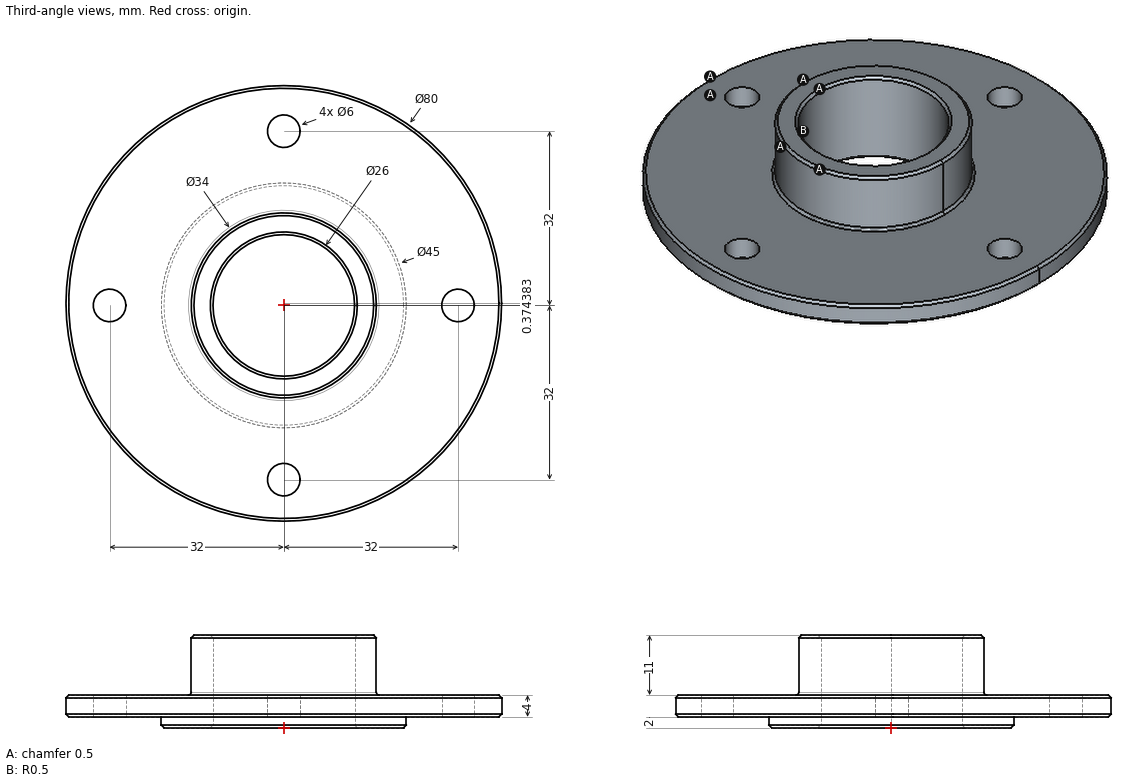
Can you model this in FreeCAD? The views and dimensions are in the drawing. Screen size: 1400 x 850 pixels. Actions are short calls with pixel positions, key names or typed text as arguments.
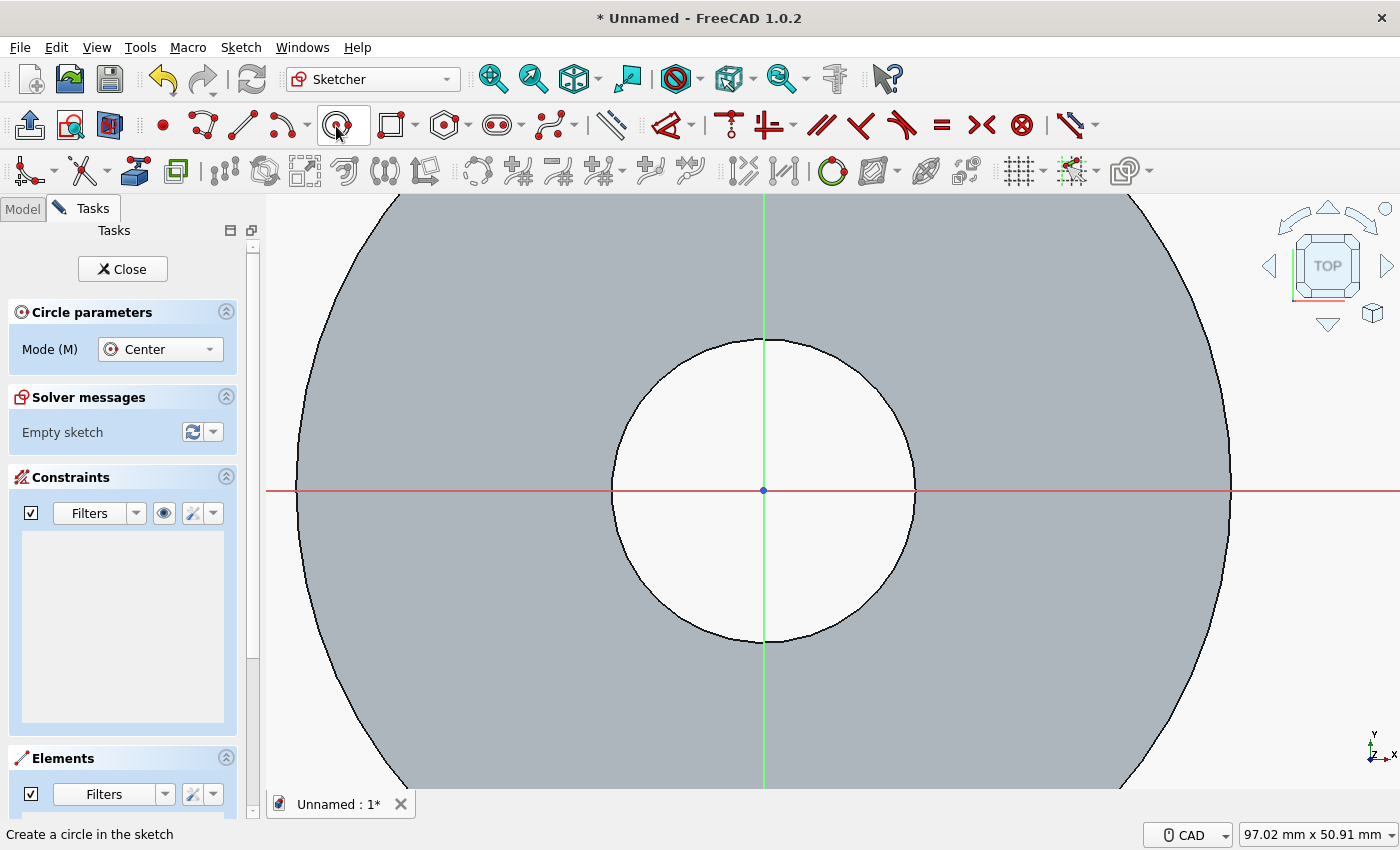
click(764, 491)
move(904, 350)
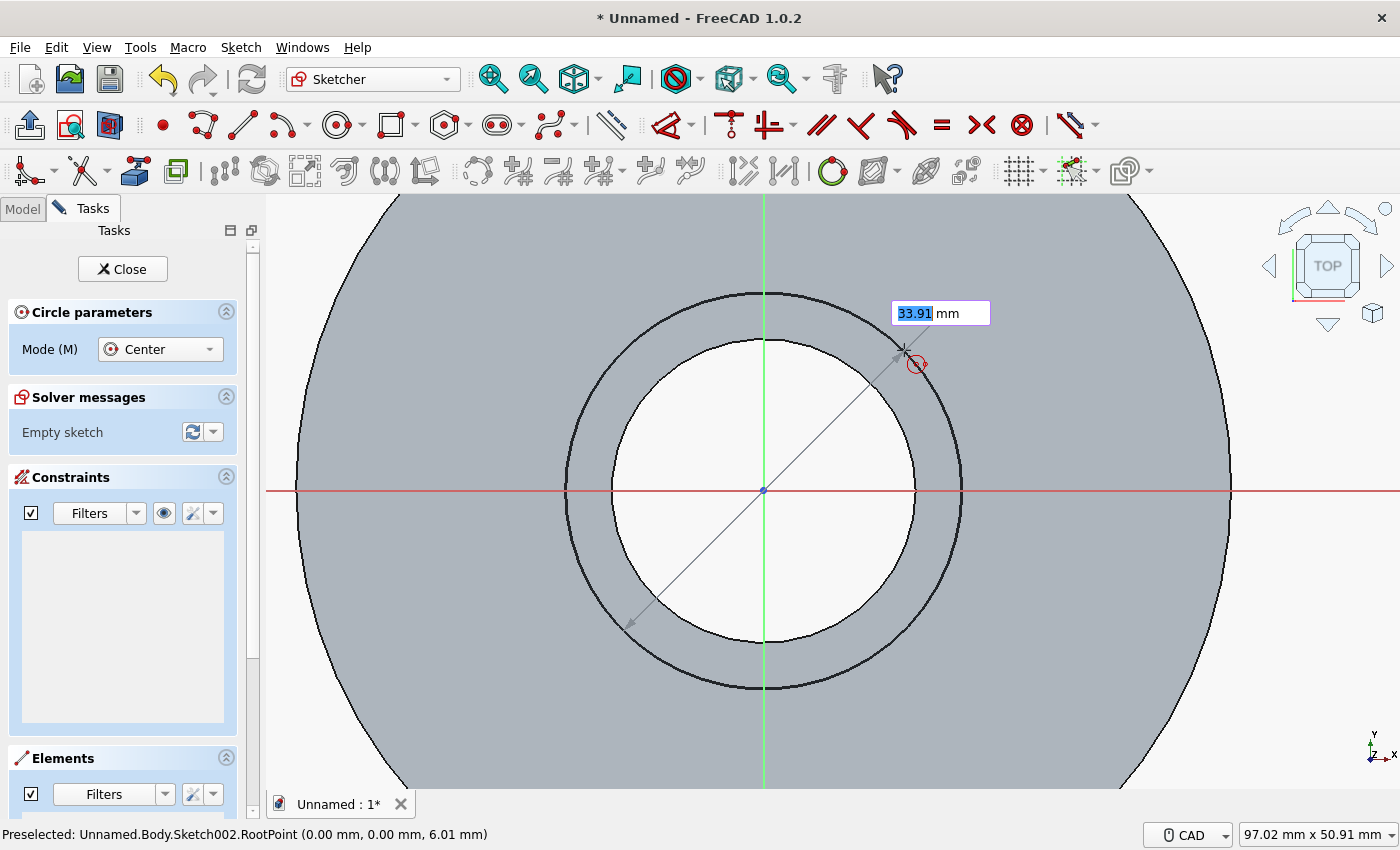
text(34)
key(Return)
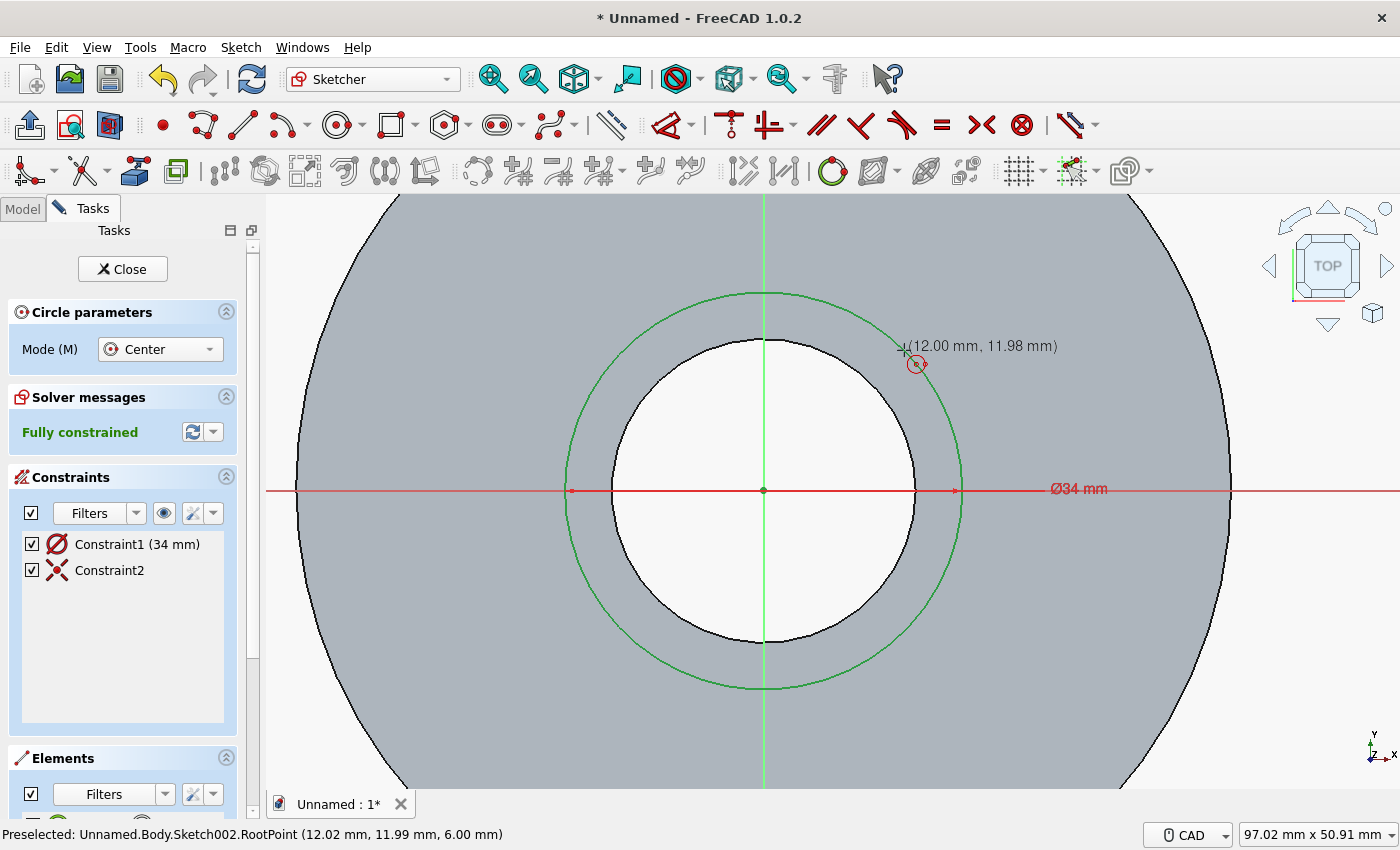
click(764, 491)
move(871, 384)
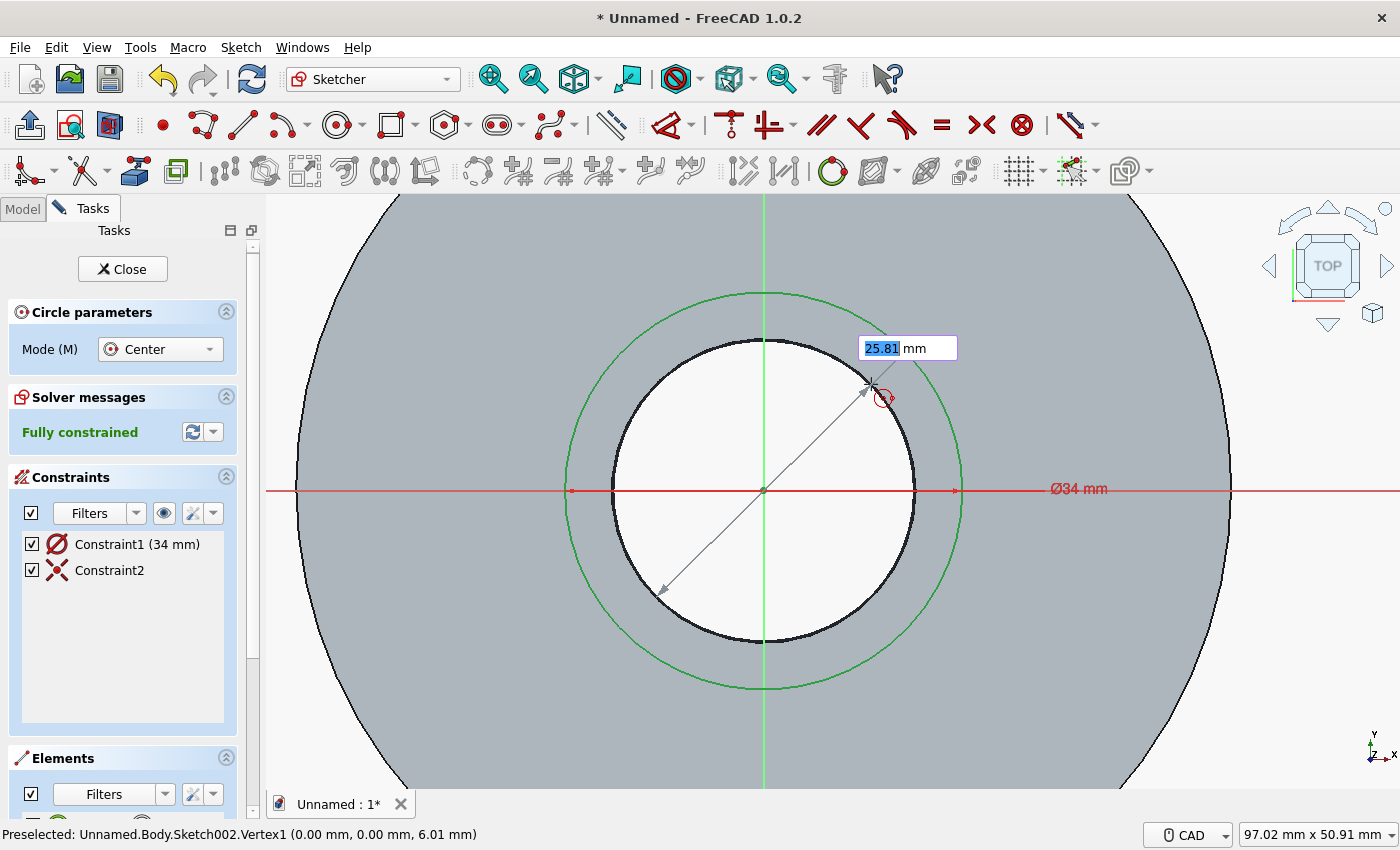
text(26)
key(Return)
key(Escape)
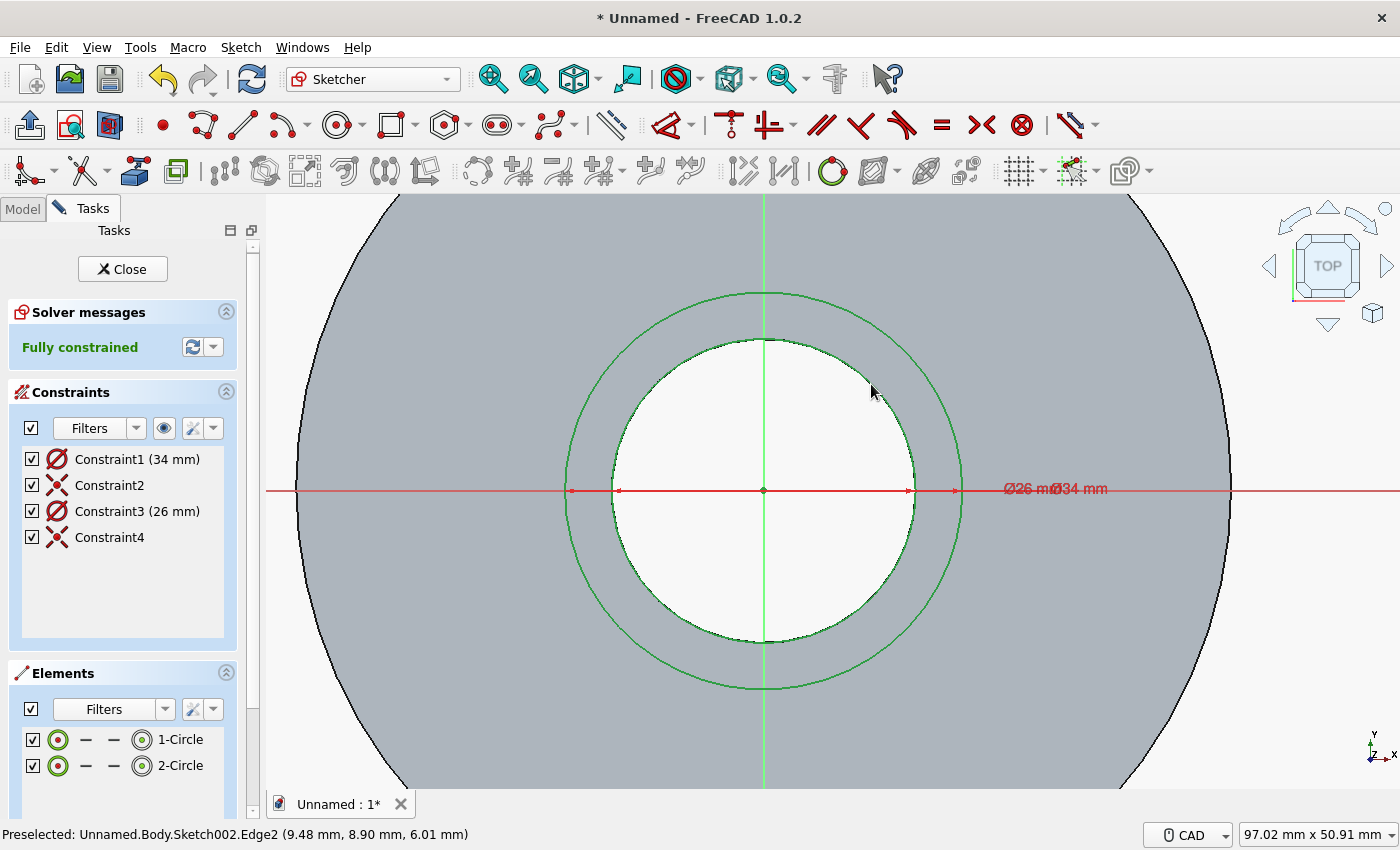
click(123, 269)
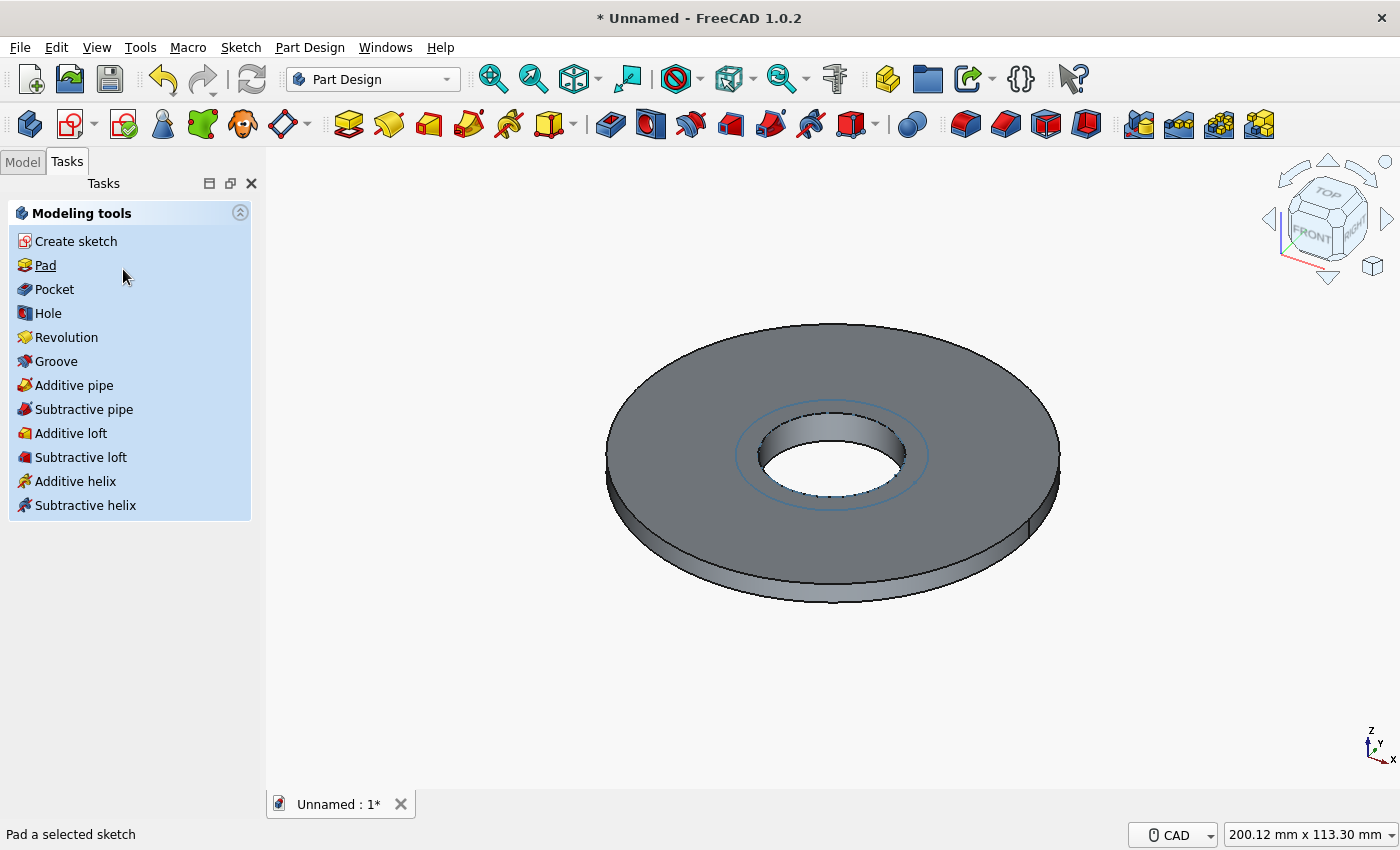
click(350, 124)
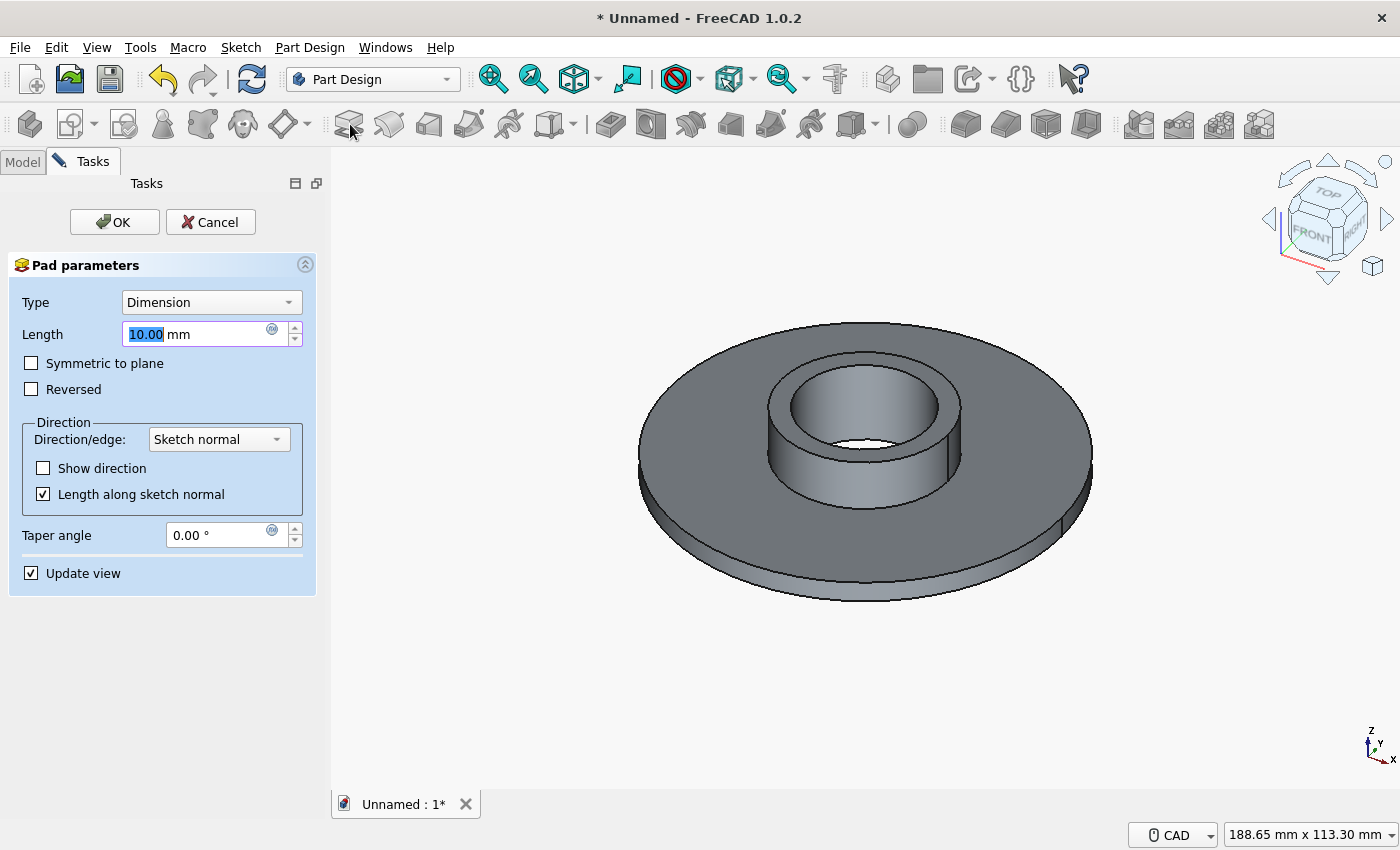
text(11)
key(Tab)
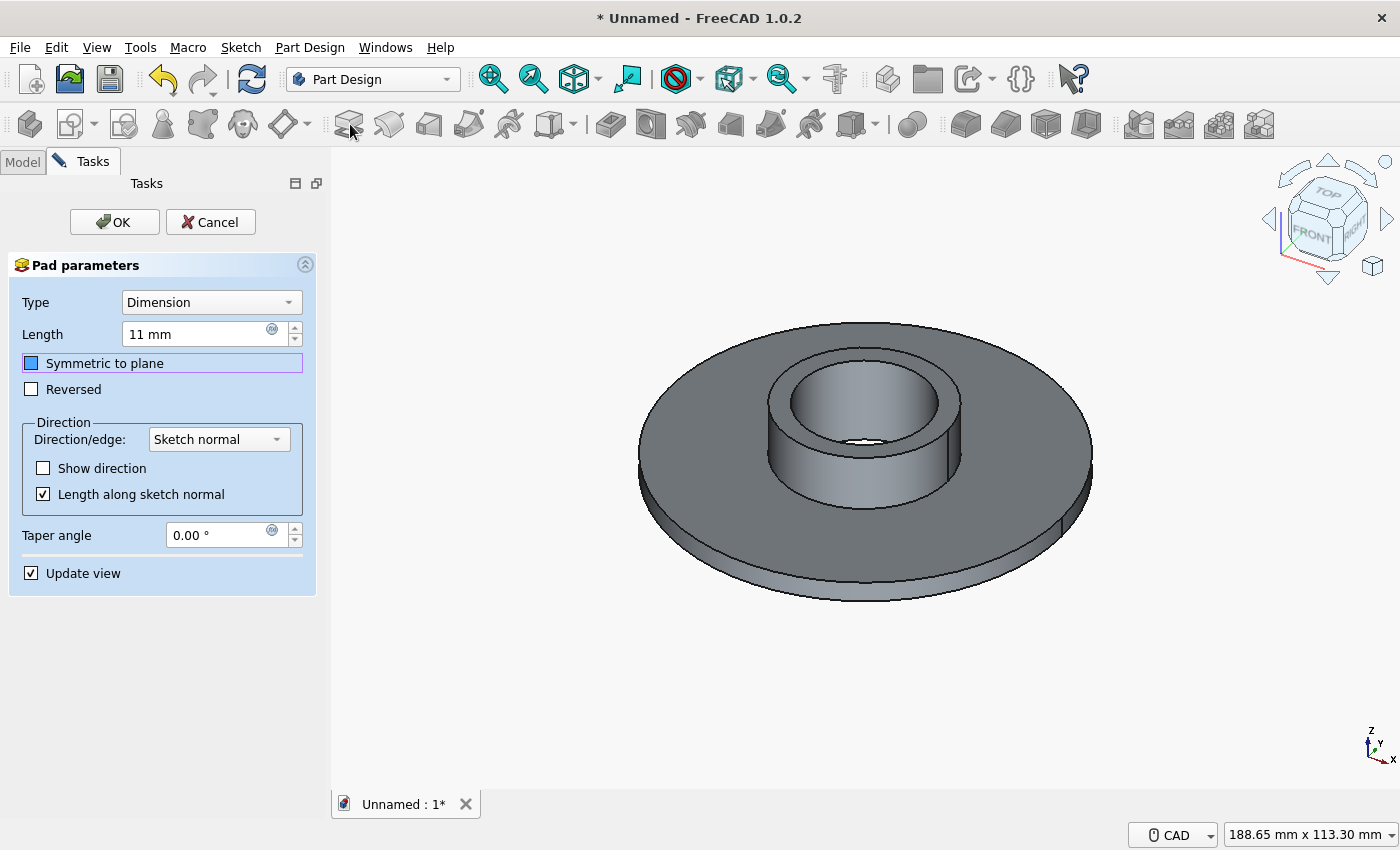
click(115, 222)